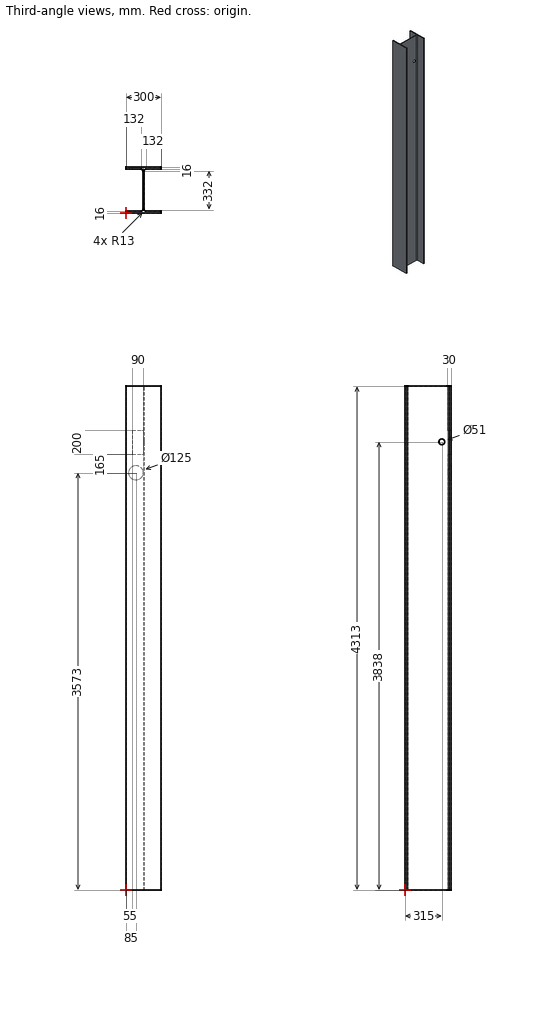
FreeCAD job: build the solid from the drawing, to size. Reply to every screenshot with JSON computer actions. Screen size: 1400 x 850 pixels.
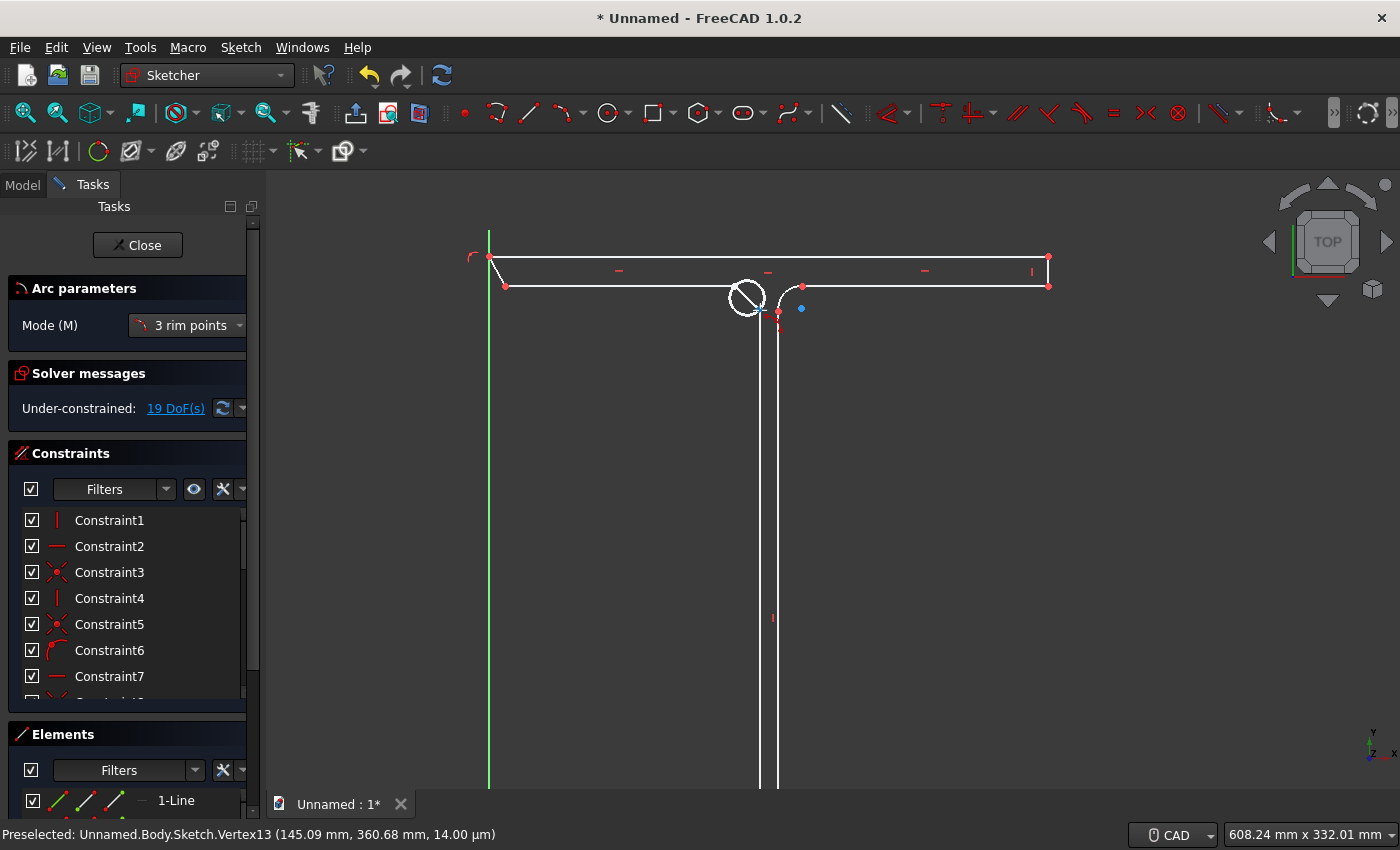
{"action": "scroll", "coordinate": [752, 292], "scroll_direction": "up", "scroll_amount": 5}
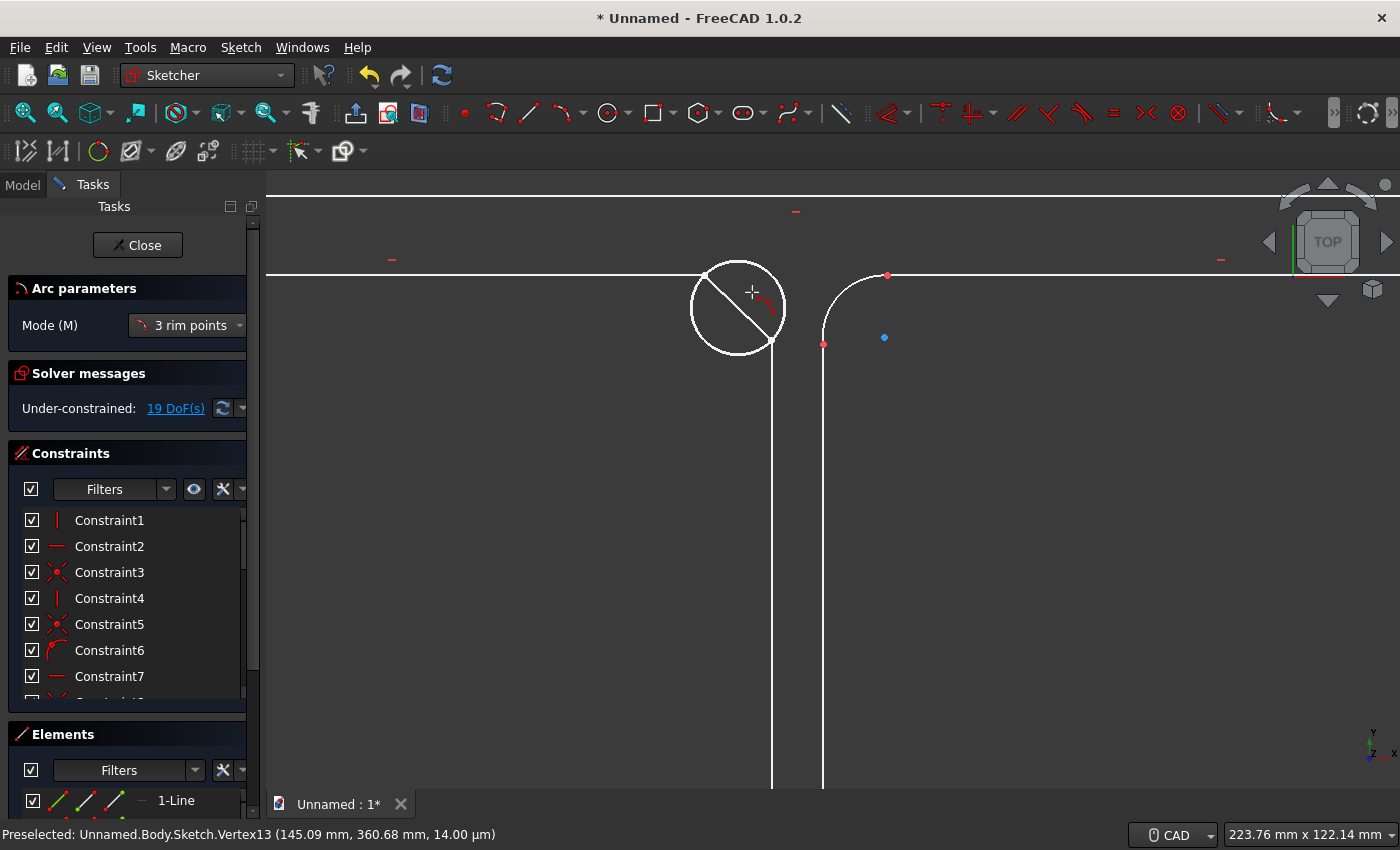
{"action": "left_click", "coordinate": [752, 292]}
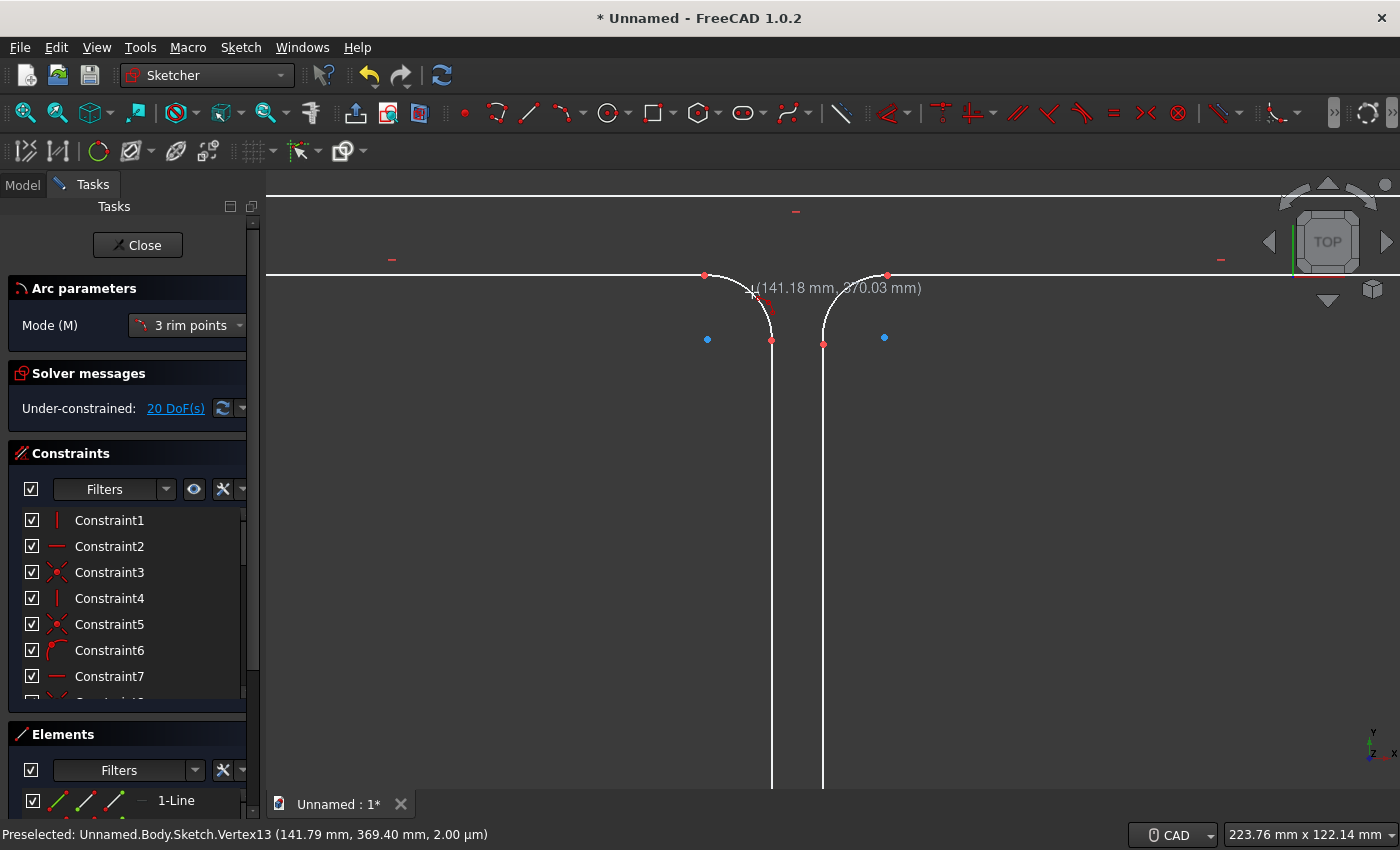
{"action": "scroll", "coordinate": [756, 302], "scroll_direction": "down", "scroll_amount": 8}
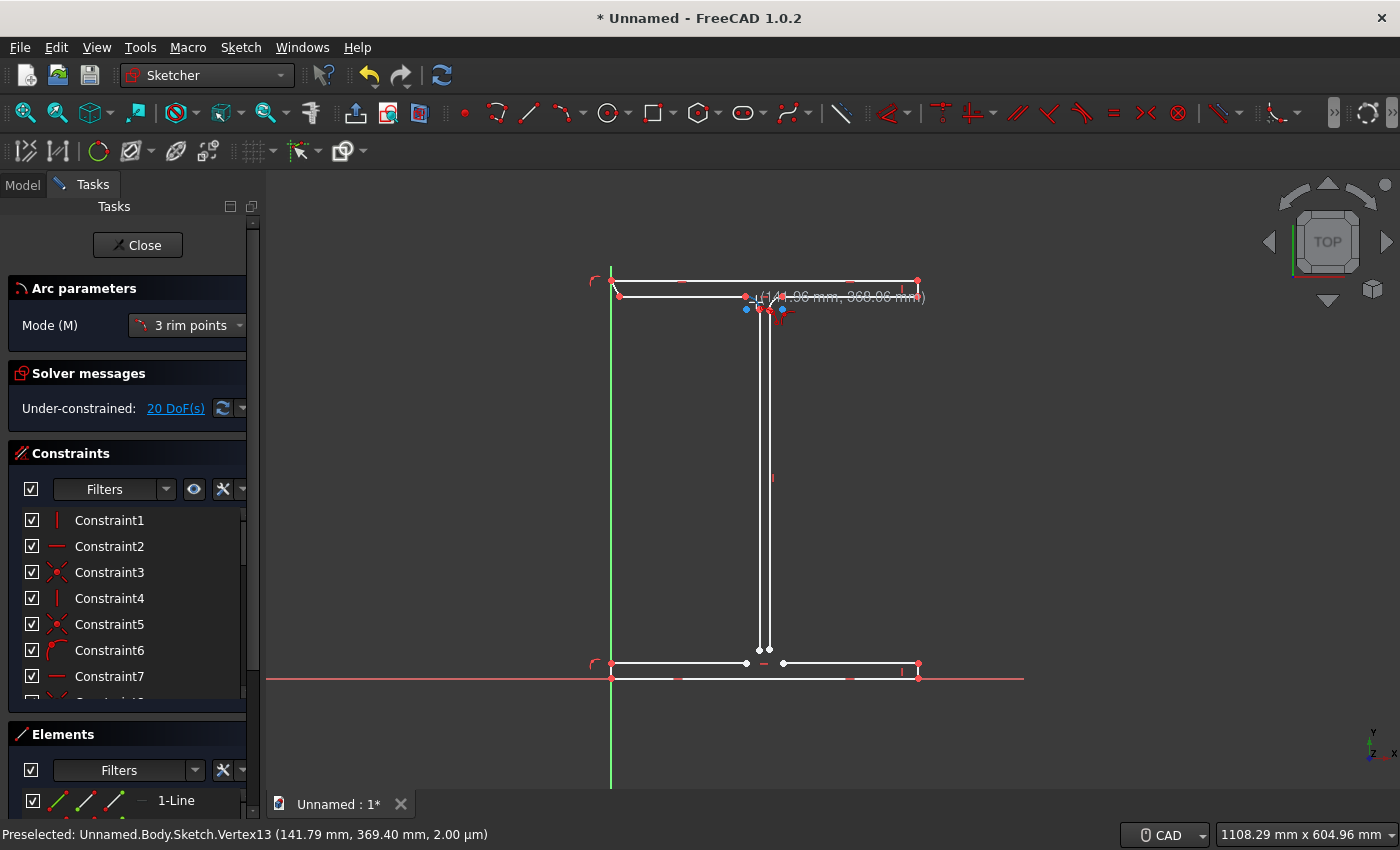
{"action": "scroll", "coordinate": [759, 649], "scroll_direction": "up", "scroll_amount": 3}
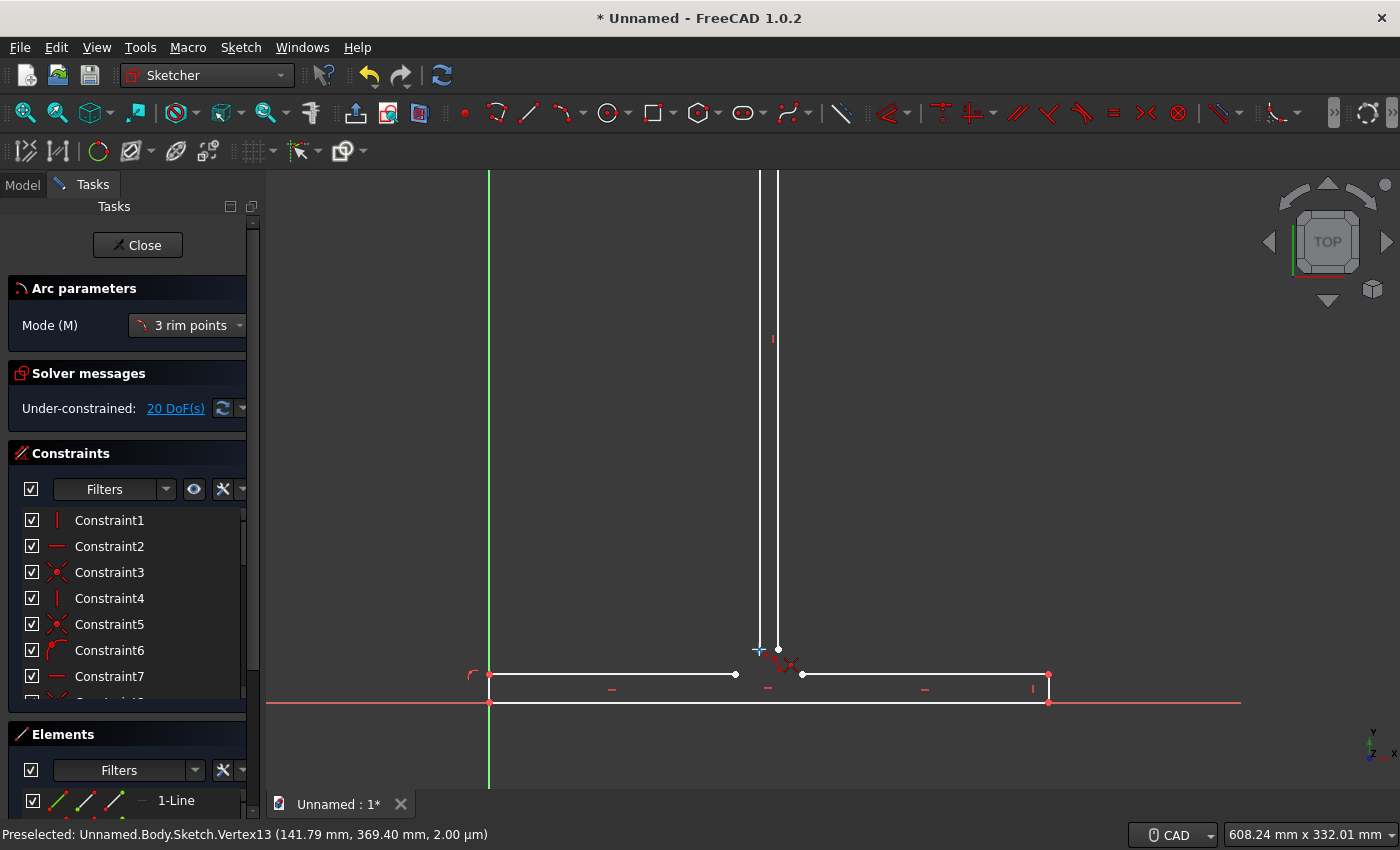
{"action": "left_click", "coordinate": [760, 650]}
{"action": "left_click", "coordinate": [736, 674]}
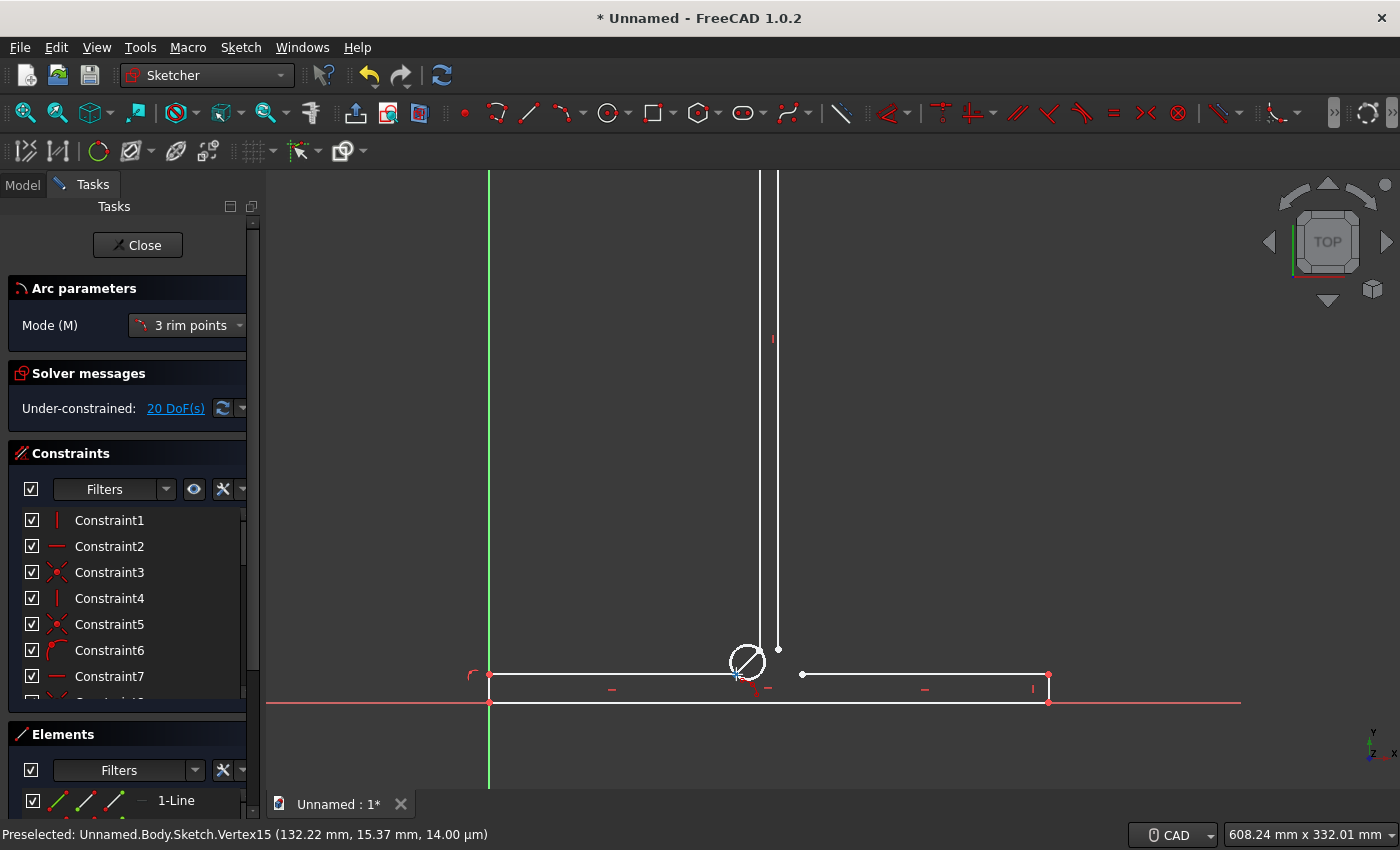
{"action": "scroll", "coordinate": [752, 666], "scroll_direction": "up", "scroll_amount": 5}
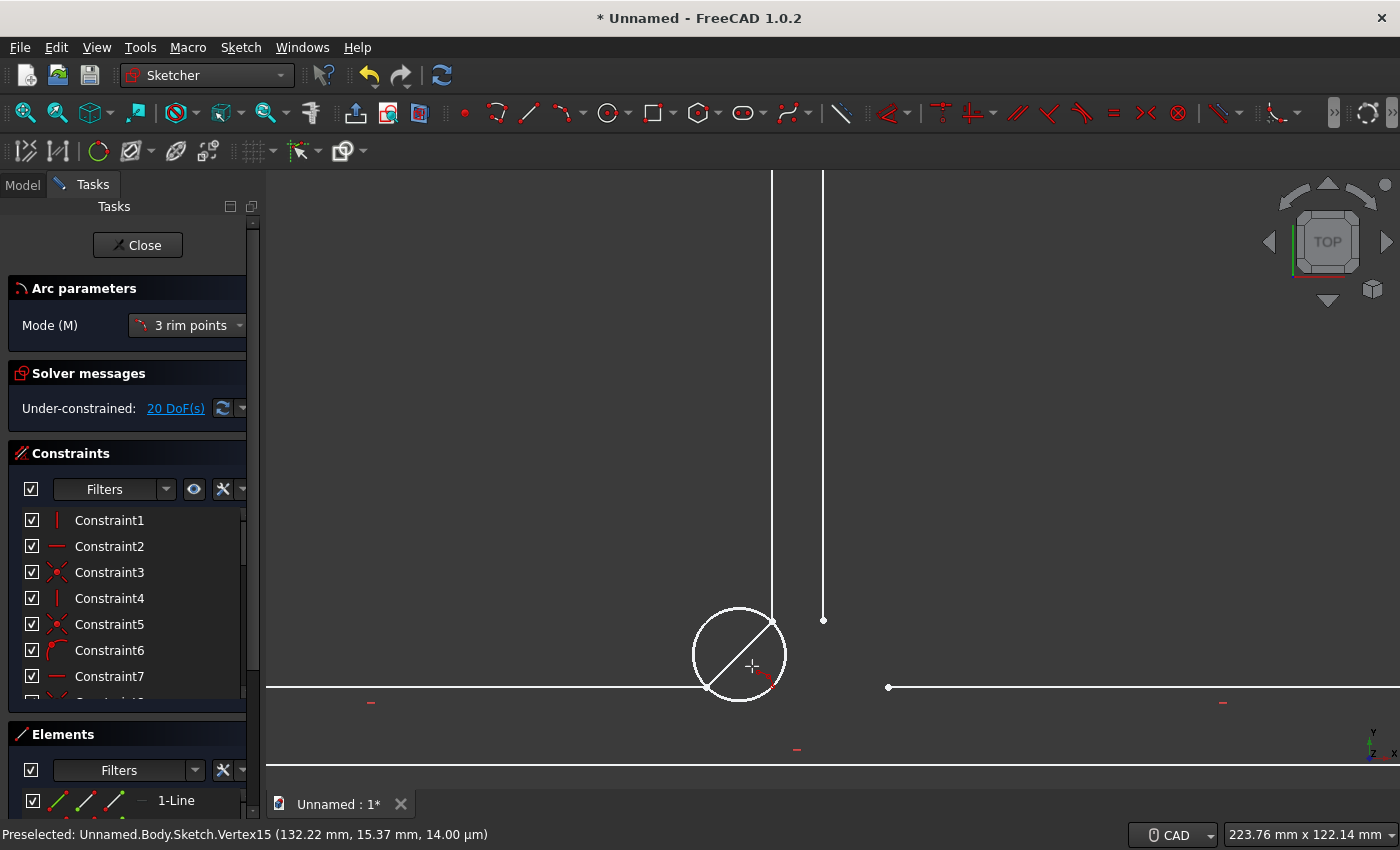
{"action": "left_click", "coordinate": [752, 665]}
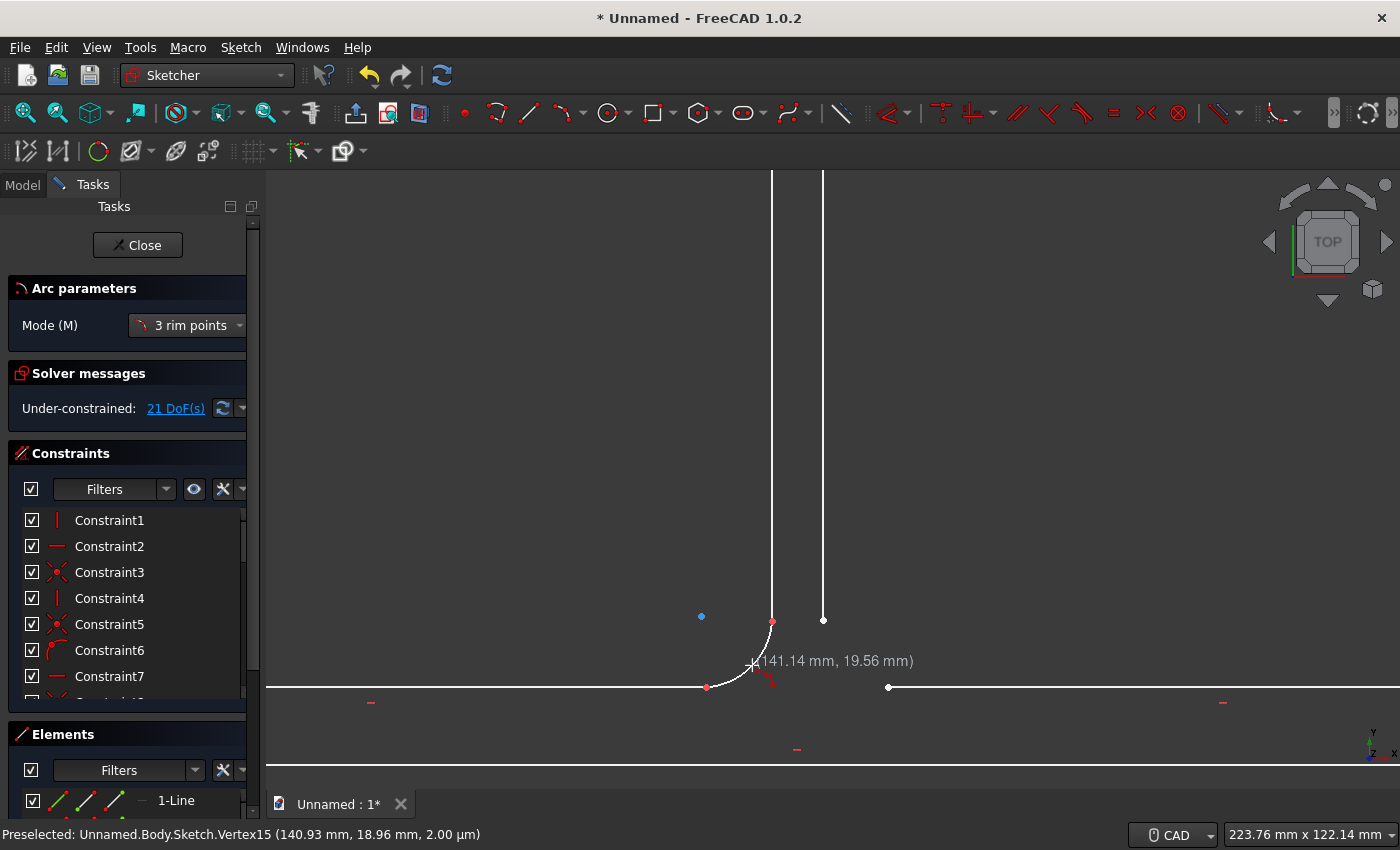
{"action": "scroll", "coordinate": [756, 657], "scroll_direction": "down", "scroll_amount": 8}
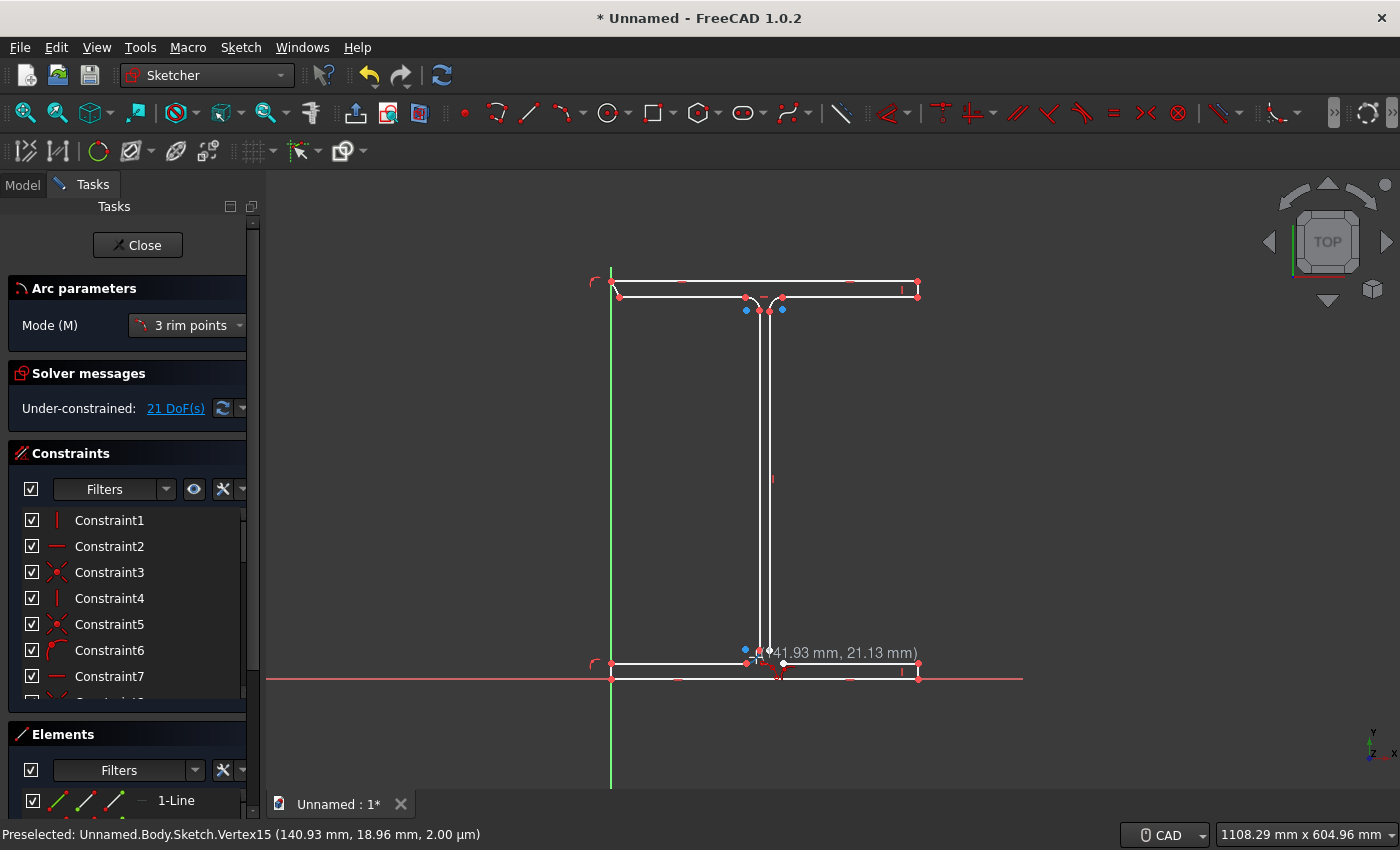
{"action": "left_click", "coordinate": [783, 664]}